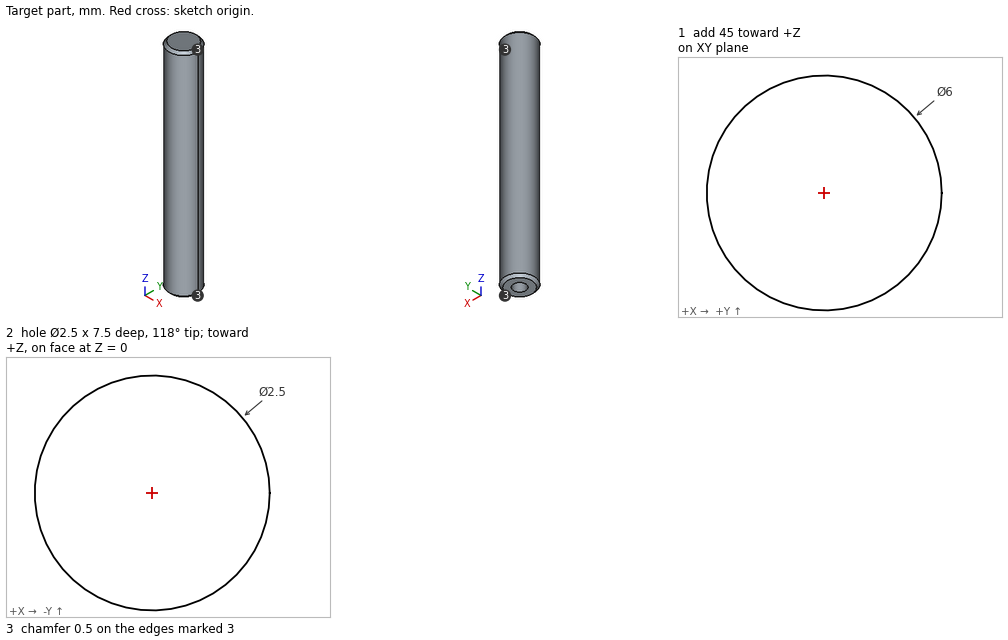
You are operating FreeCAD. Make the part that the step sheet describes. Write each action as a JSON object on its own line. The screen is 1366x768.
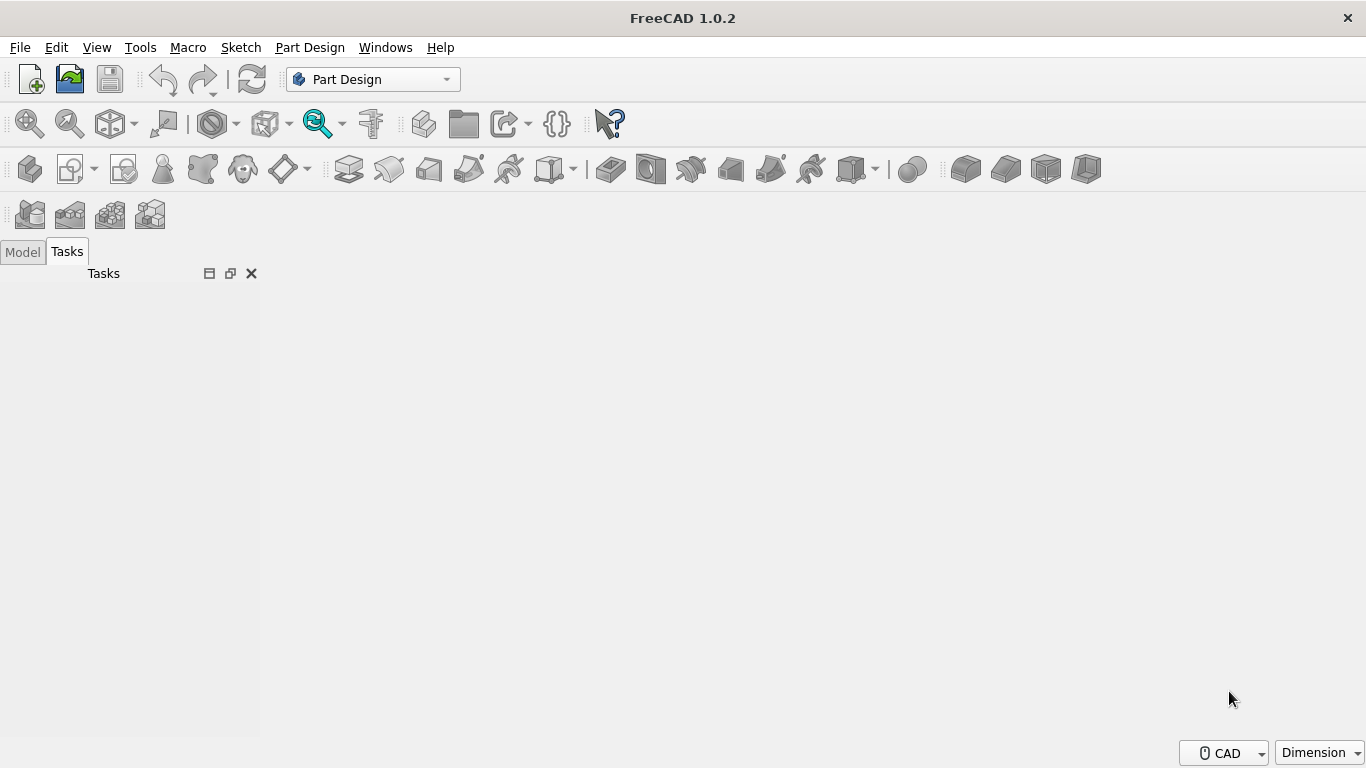
{"action": "left_click", "coordinate": [30, 80]}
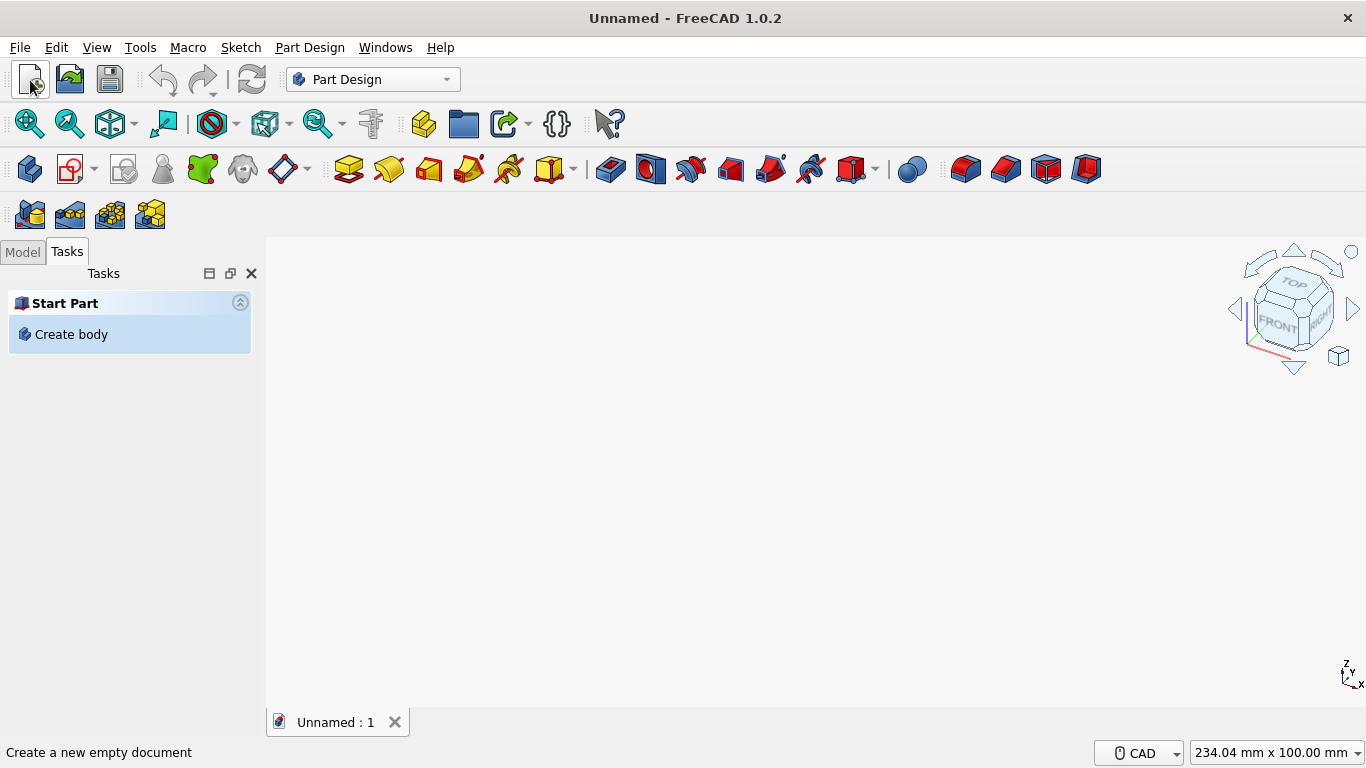
{"action": "left_click", "coordinate": [70, 170]}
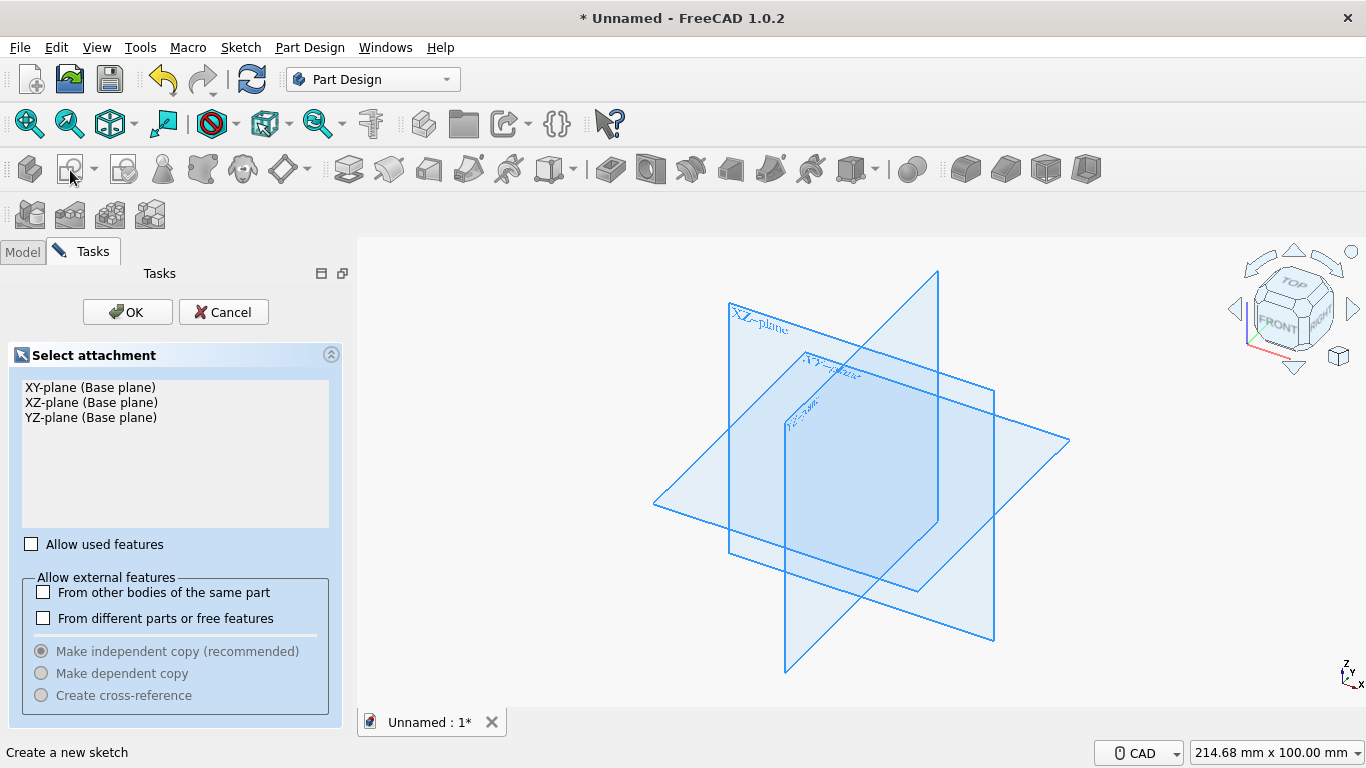
{"action": "left_click", "coordinate": [82, 388]}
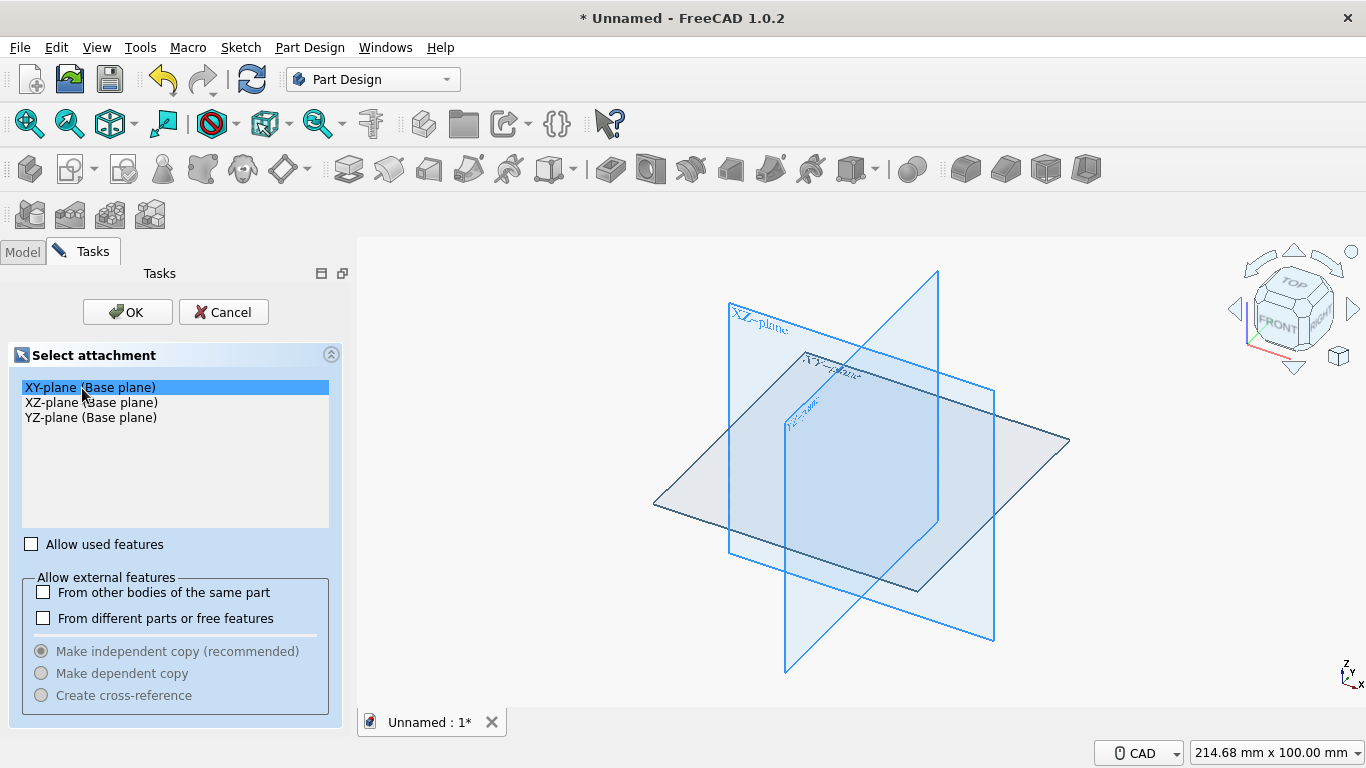
{"action": "left_click", "coordinate": [128, 312]}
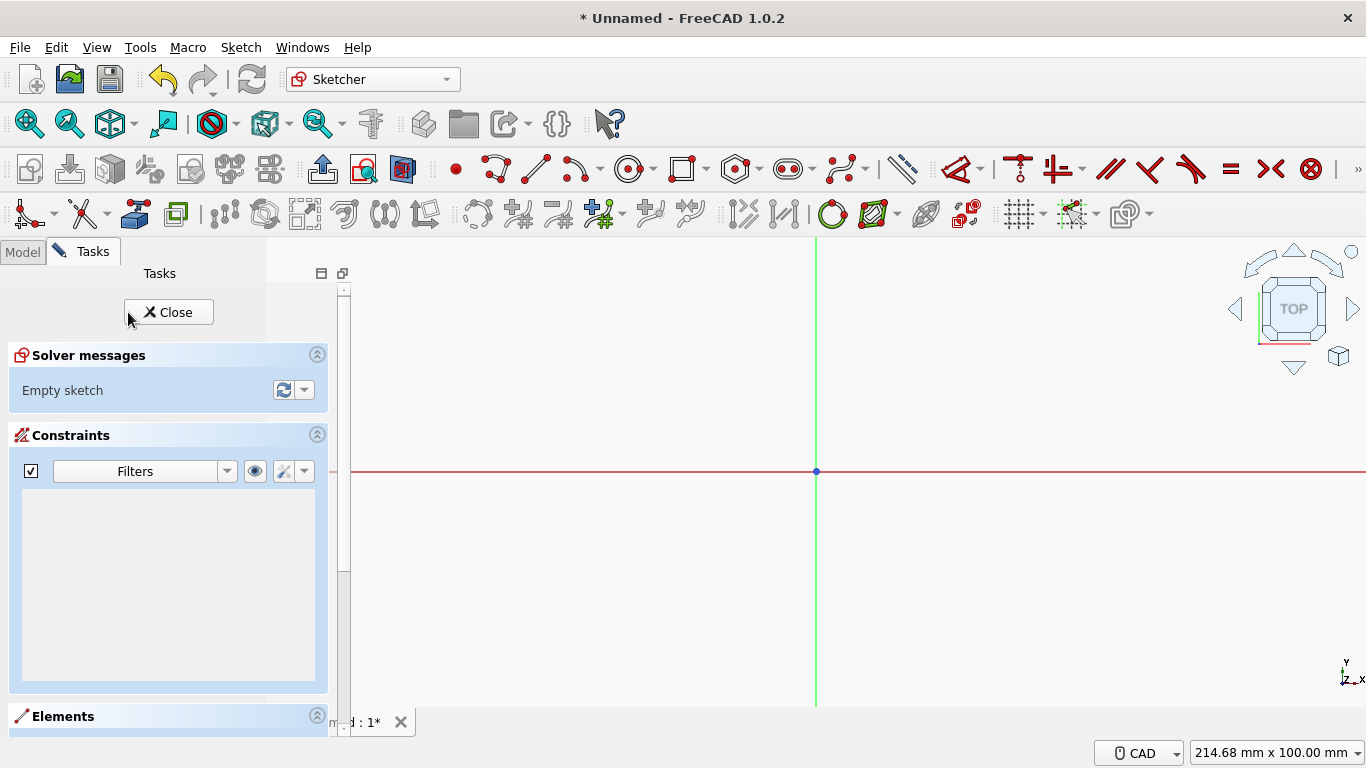
{"action": "scroll", "coordinate": [823, 472], "scroll_direction": "up", "scroll_amount": 12}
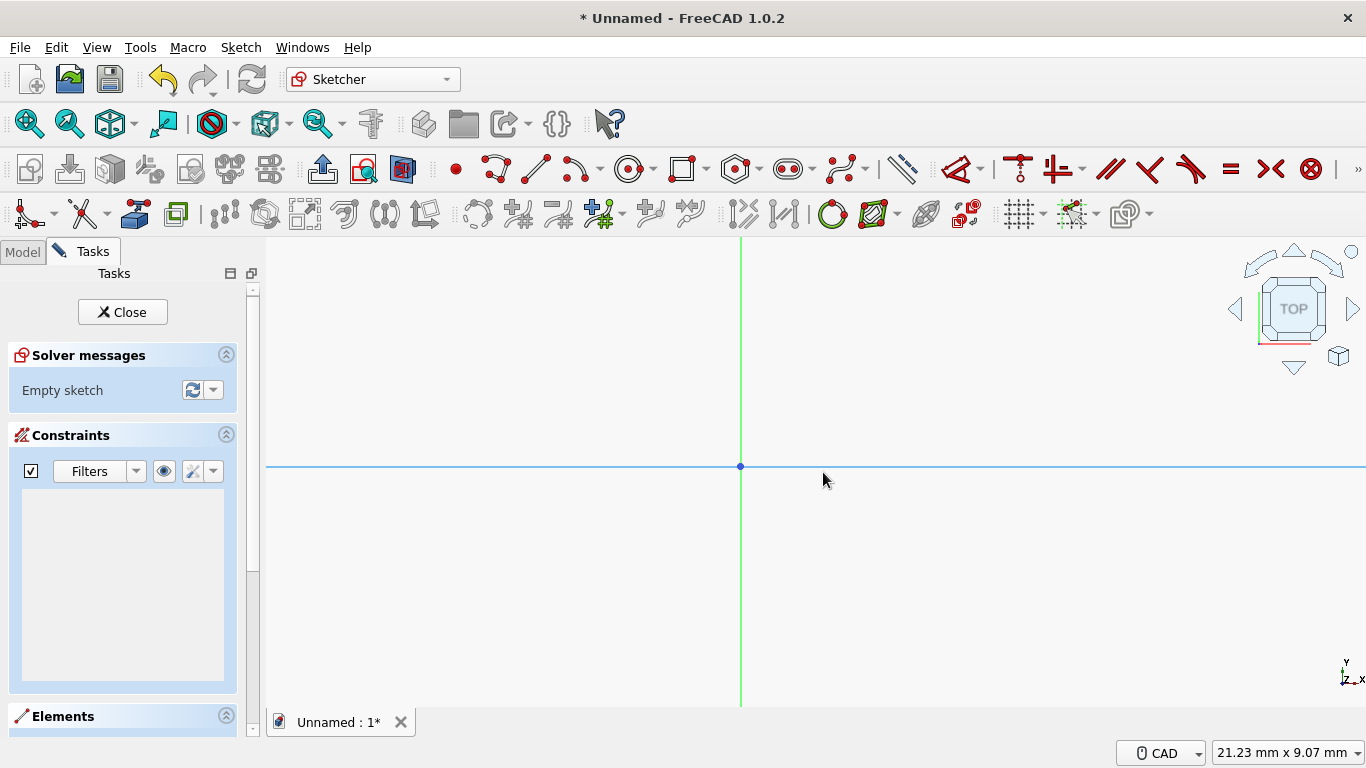
{"action": "left_click", "coordinate": [630, 170]}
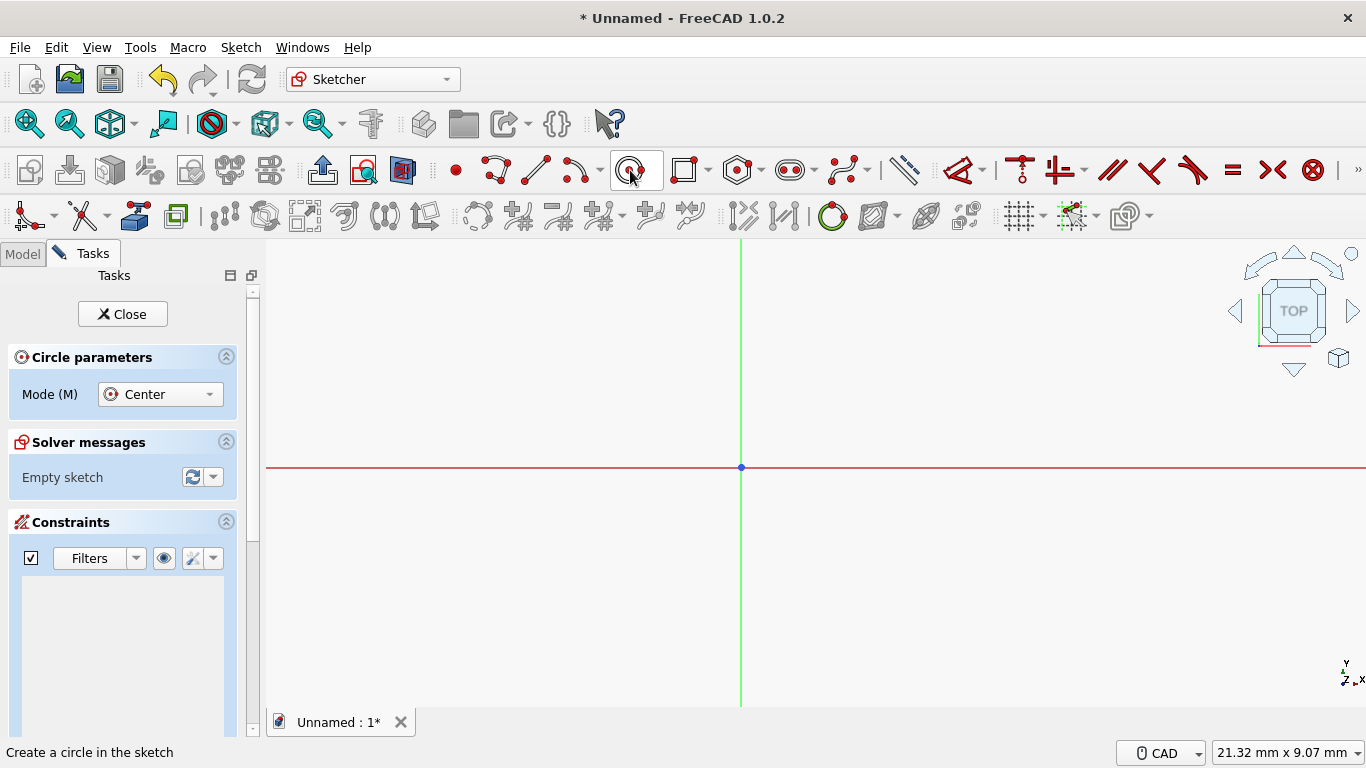
{"action": "left_click", "coordinate": [741, 468]}
{"action": "mouse_move", "coordinate": [851, 359]}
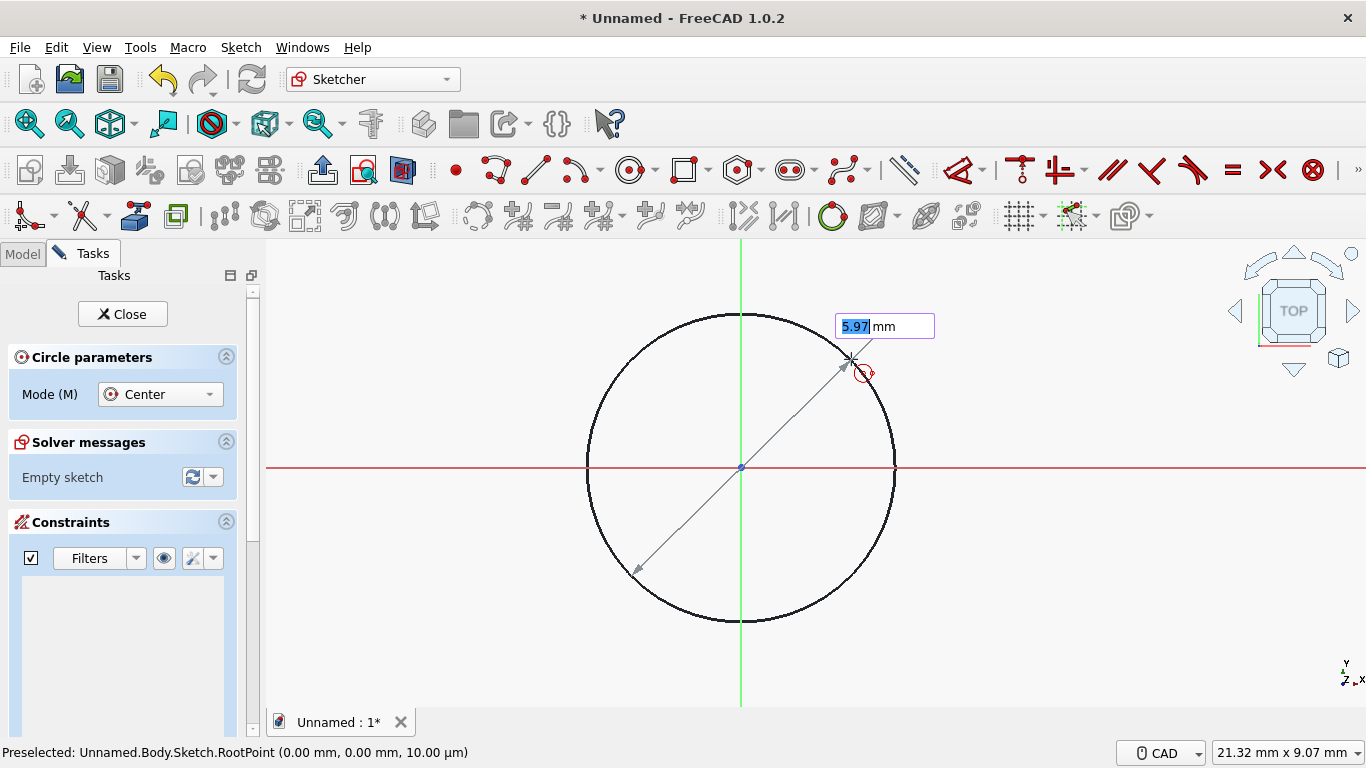
{"action": "type", "text": "6"}
{"action": "key", "text": "Return"}
{"action": "key", "text": "Escape"}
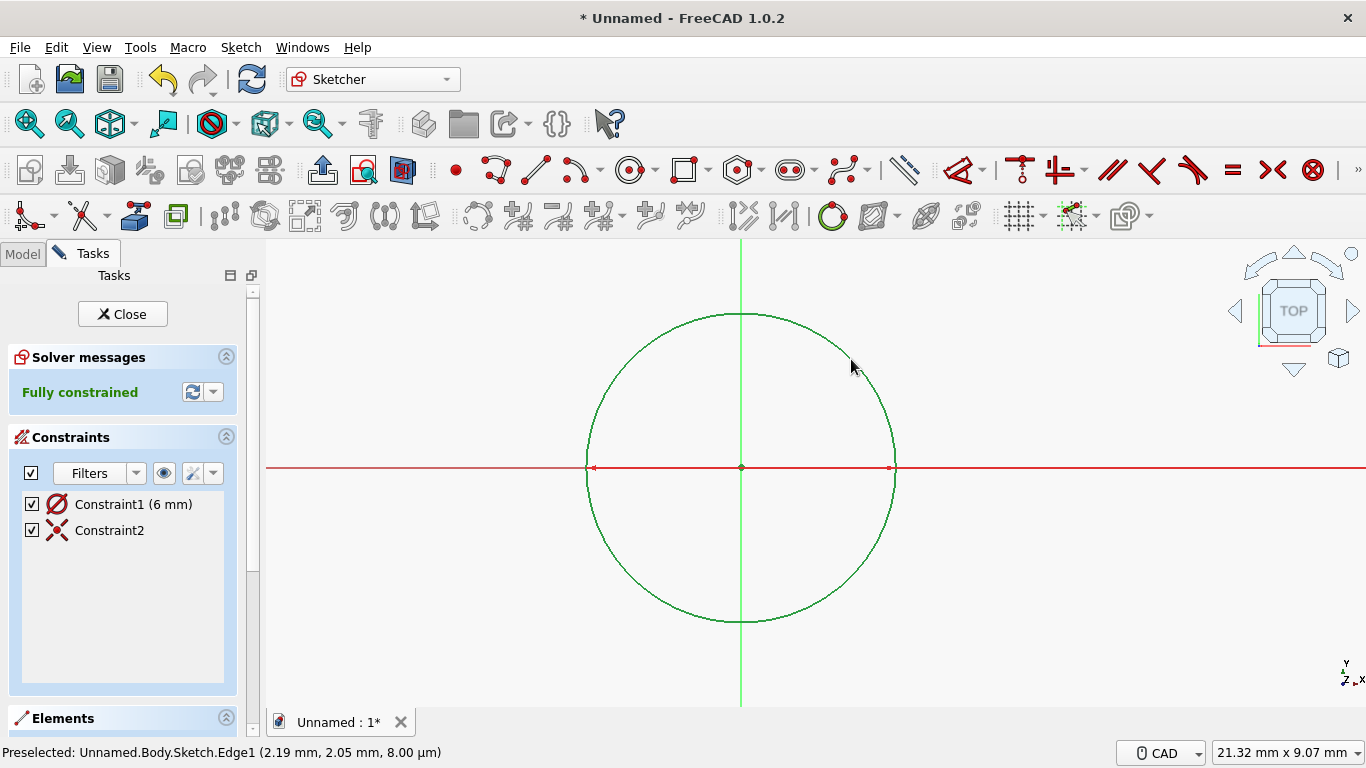
{"action": "left_click", "coordinate": [123, 314]}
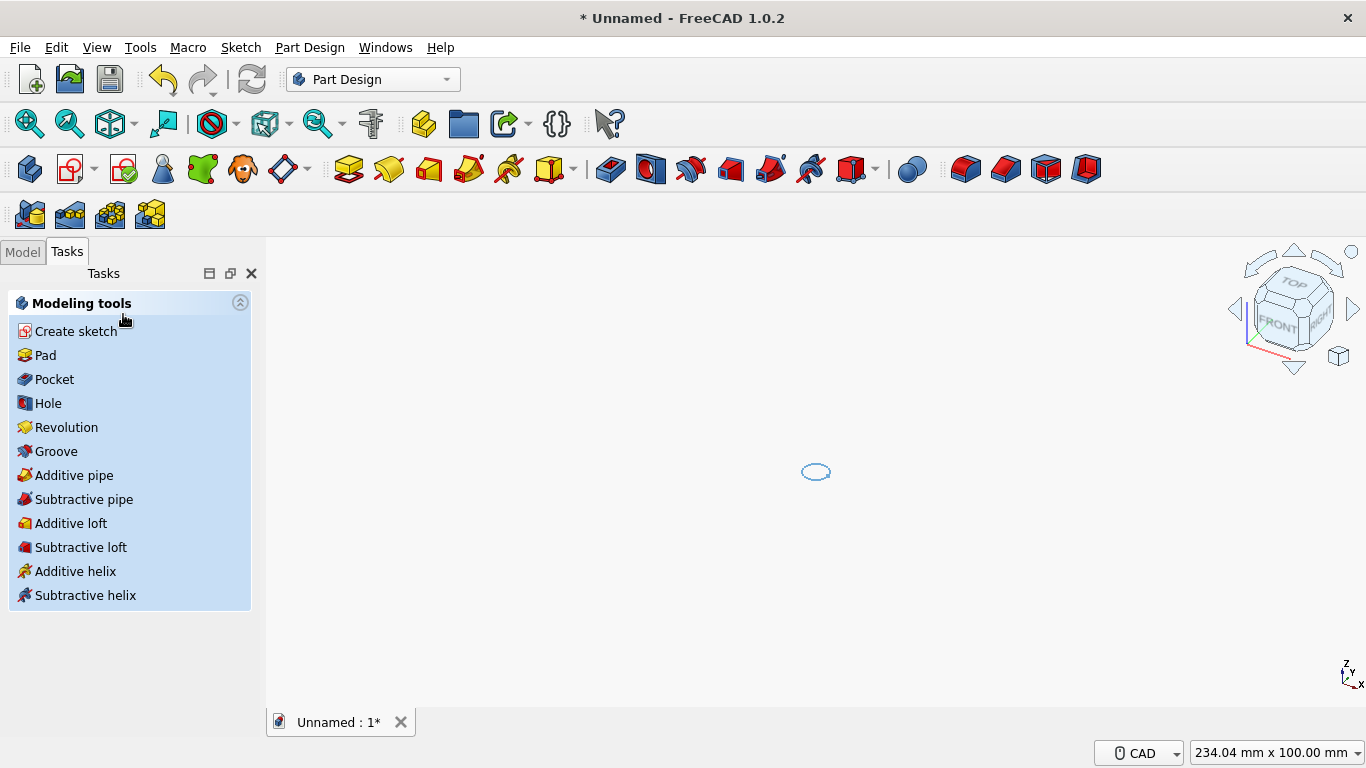
{"action": "left_click", "coordinate": [350, 170]}